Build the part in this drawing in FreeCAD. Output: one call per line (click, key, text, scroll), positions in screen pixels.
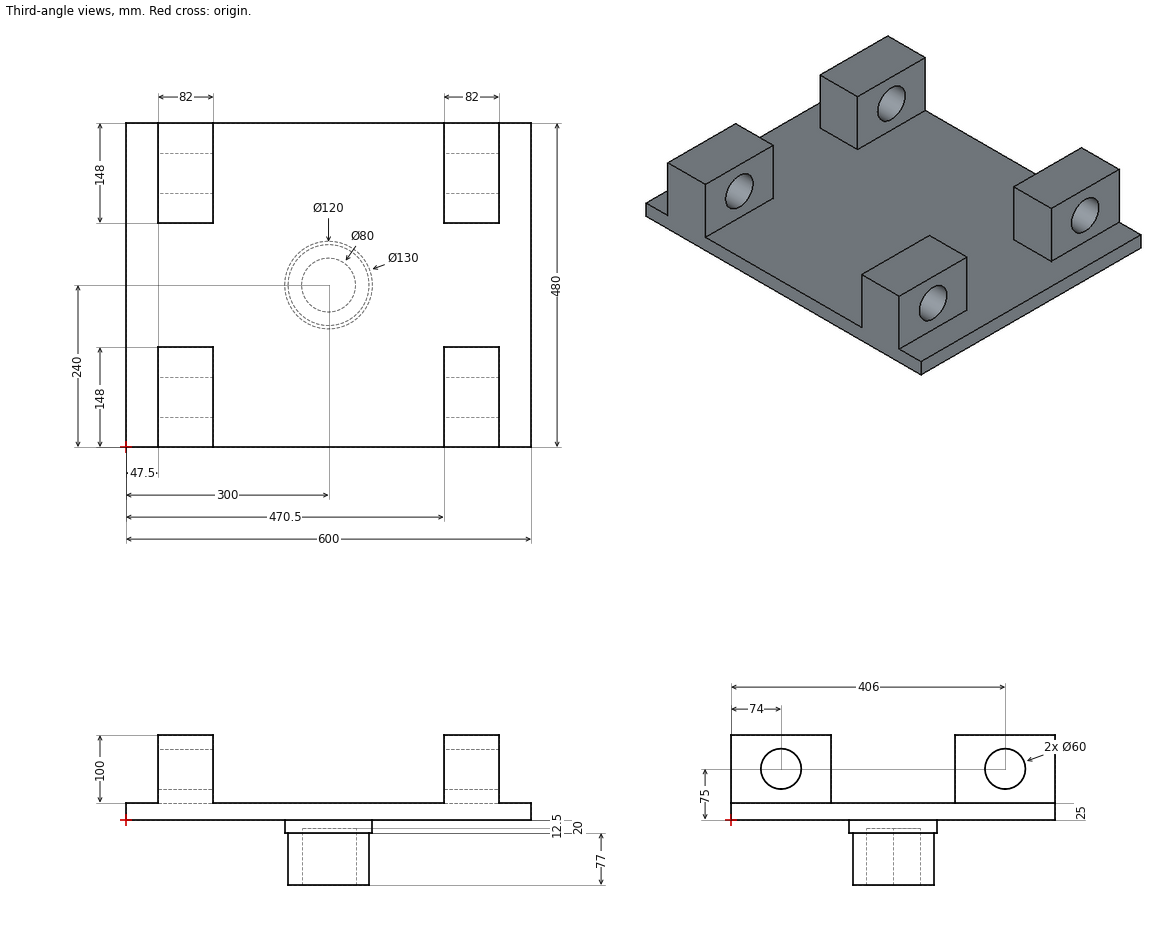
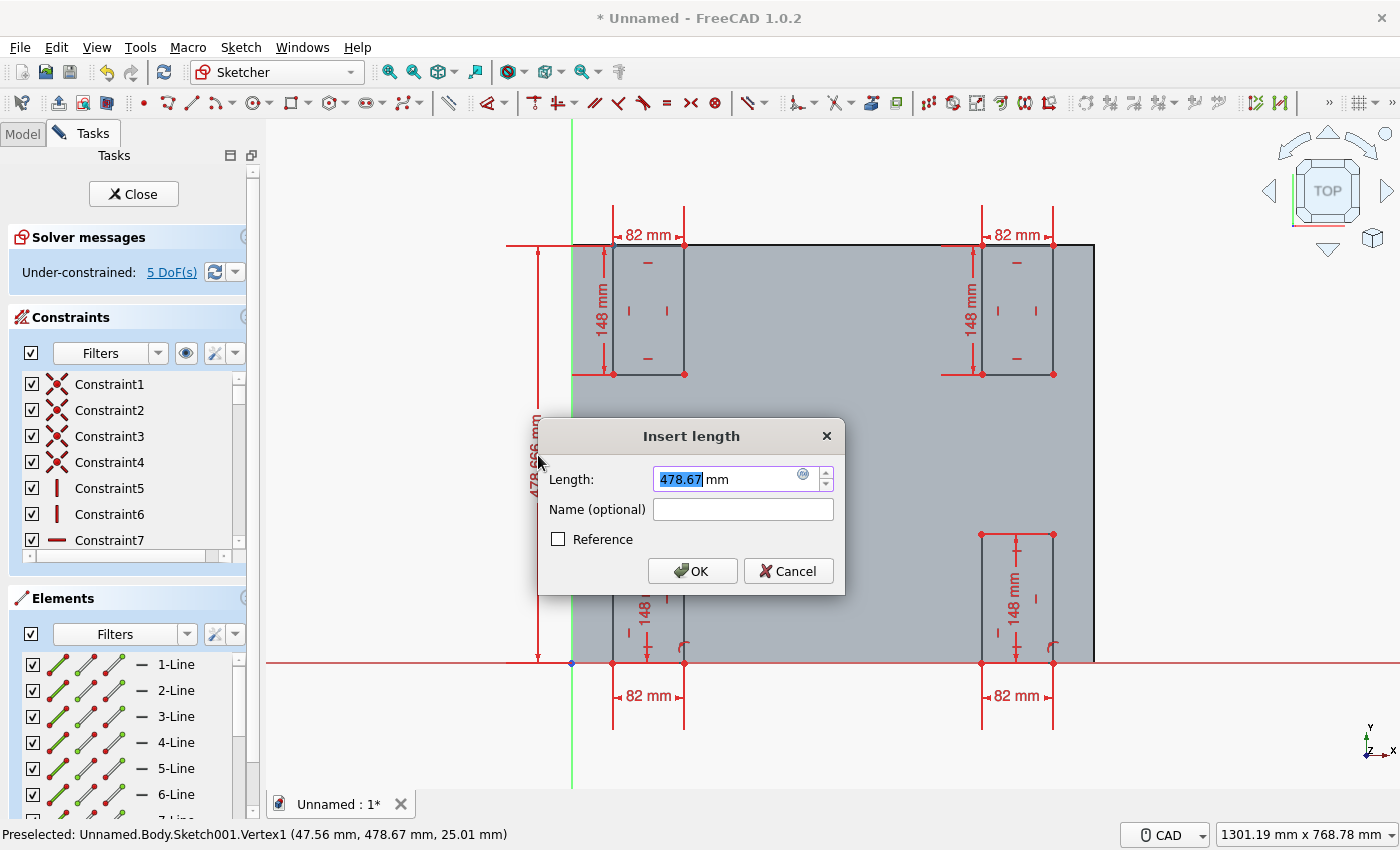
text(480)
key(Return)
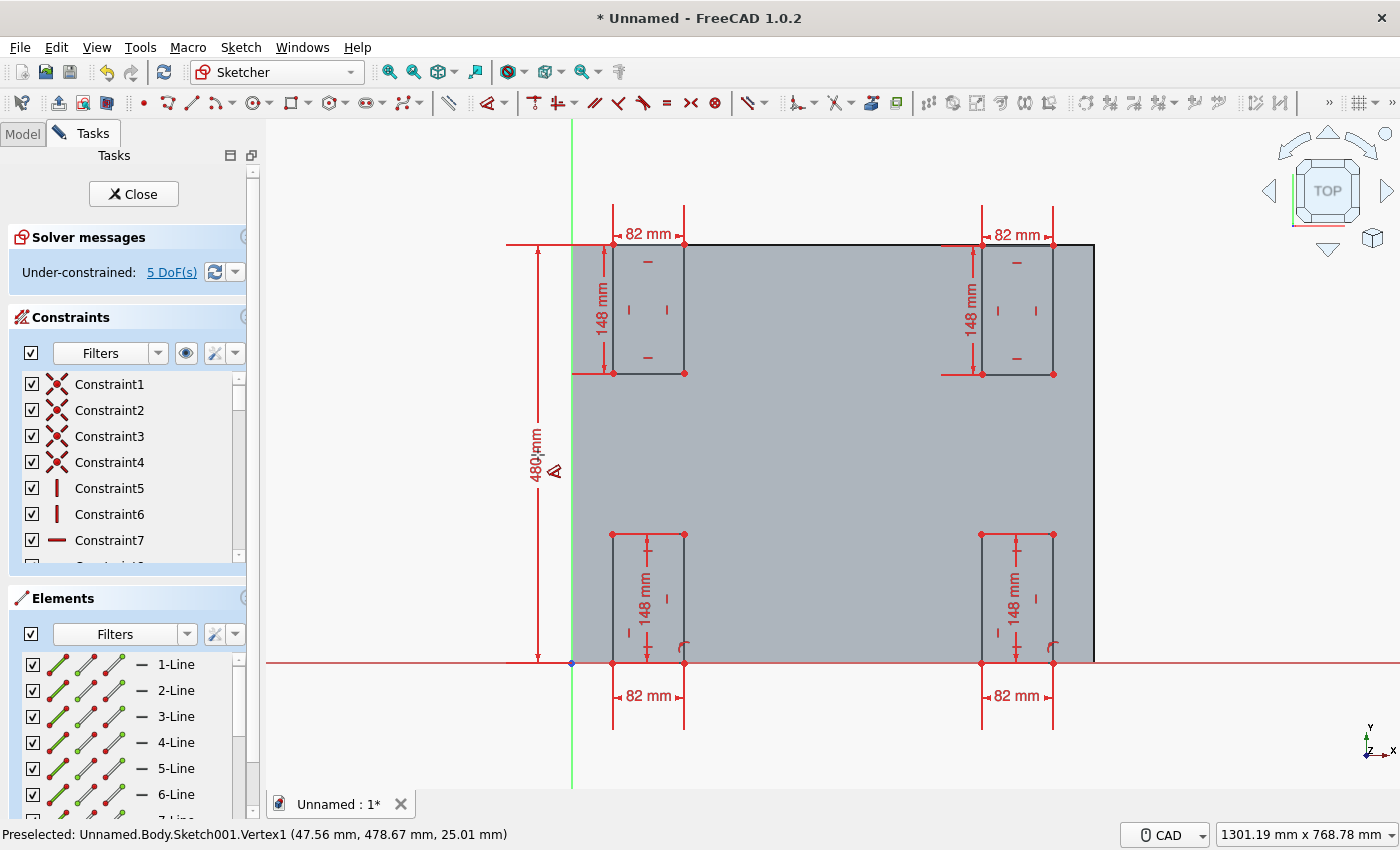
click(982, 246)
click(538, 359)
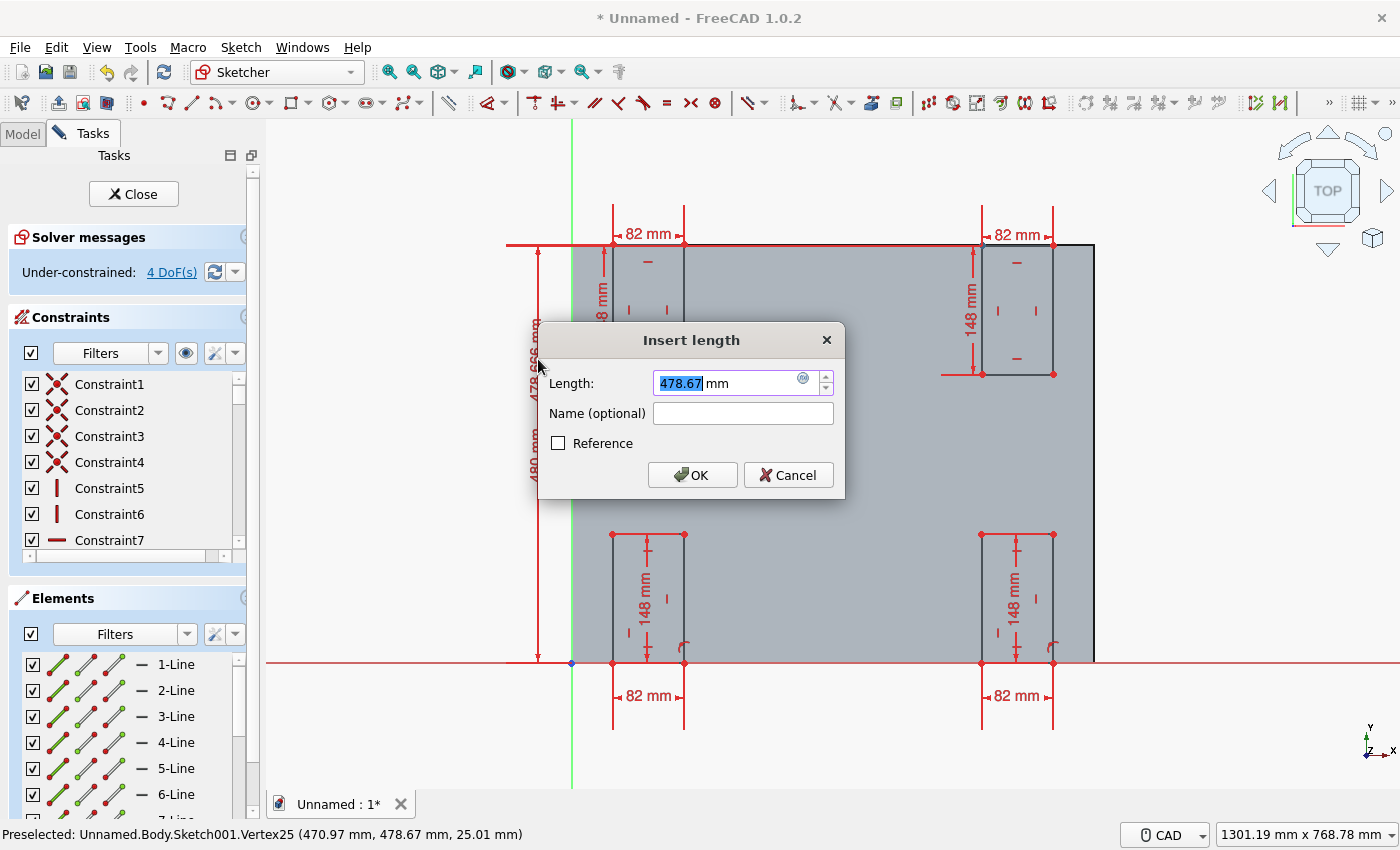
text(480)
key(Return)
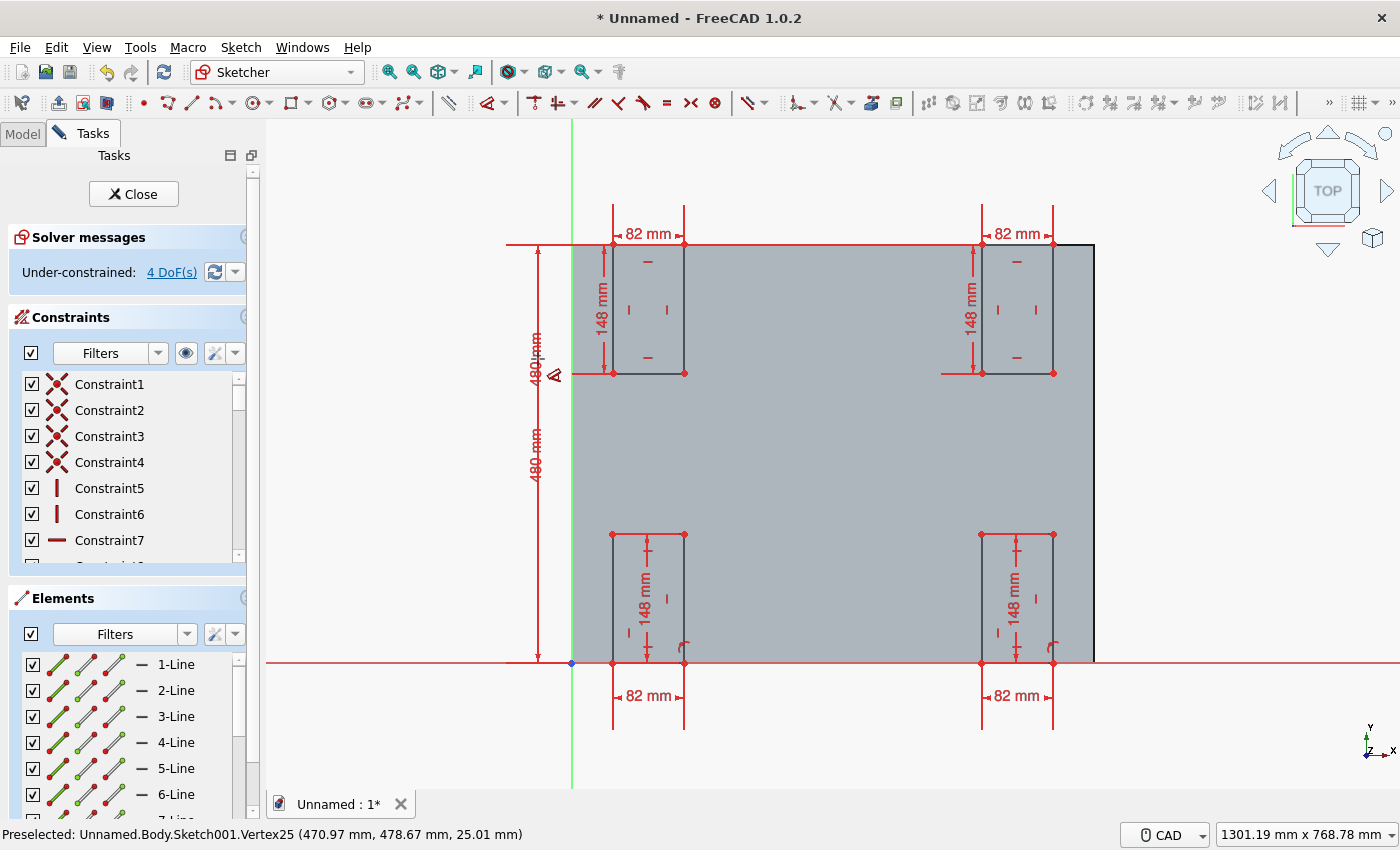
click(613, 245)
click(592, 211)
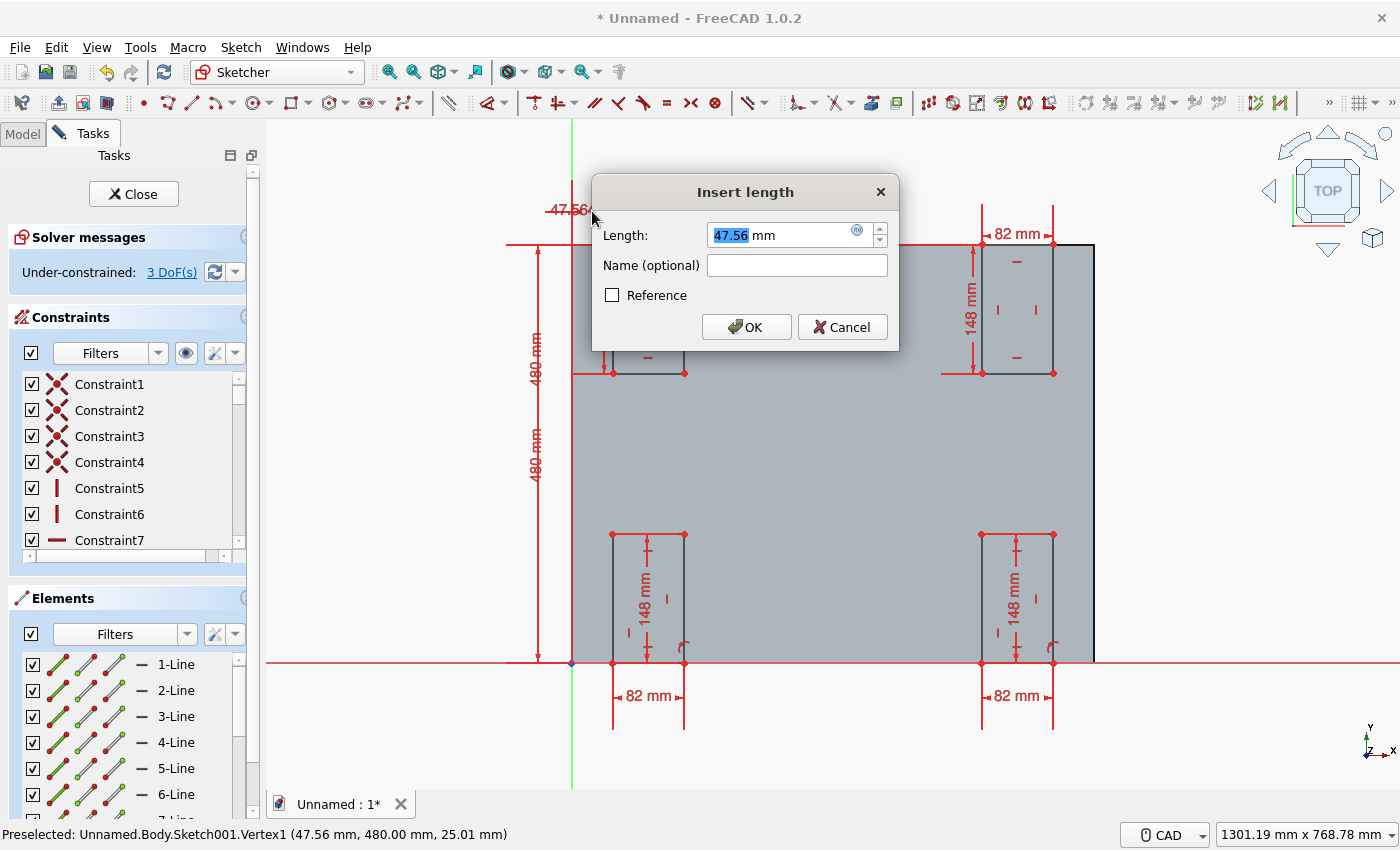
text(47.5)
key(Return)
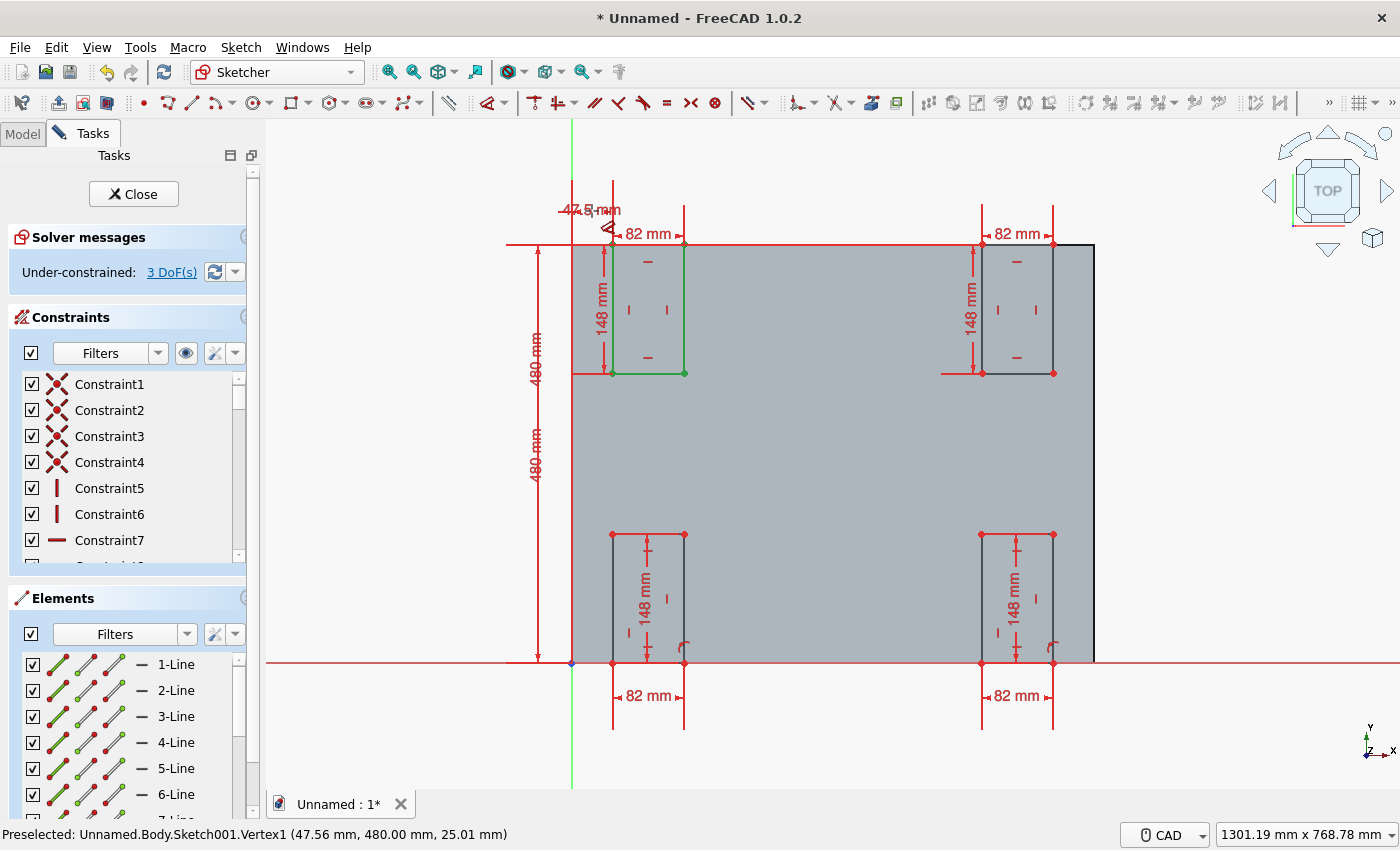
click(613, 534)
click(592, 500)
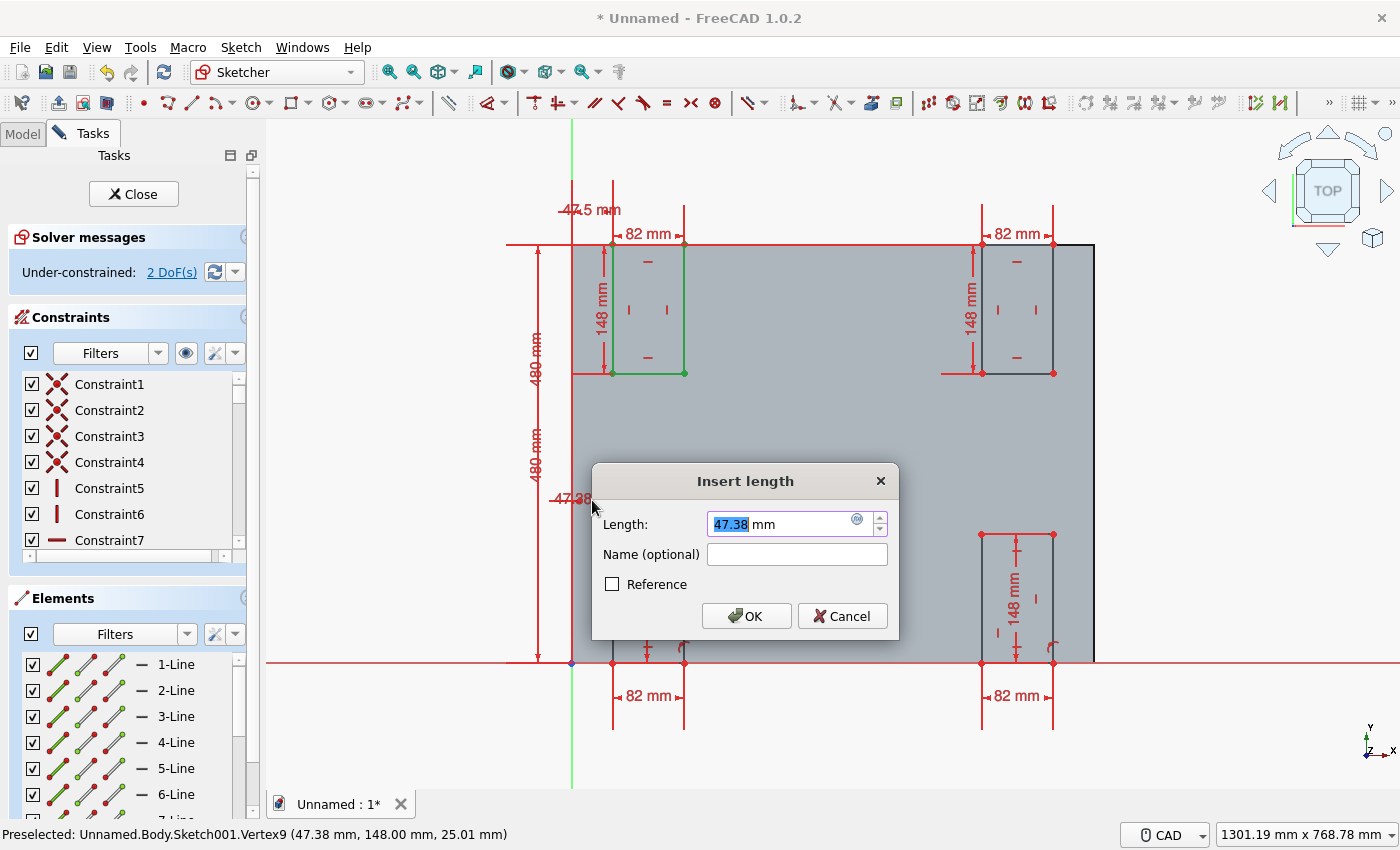
text(47.5)
key(Return)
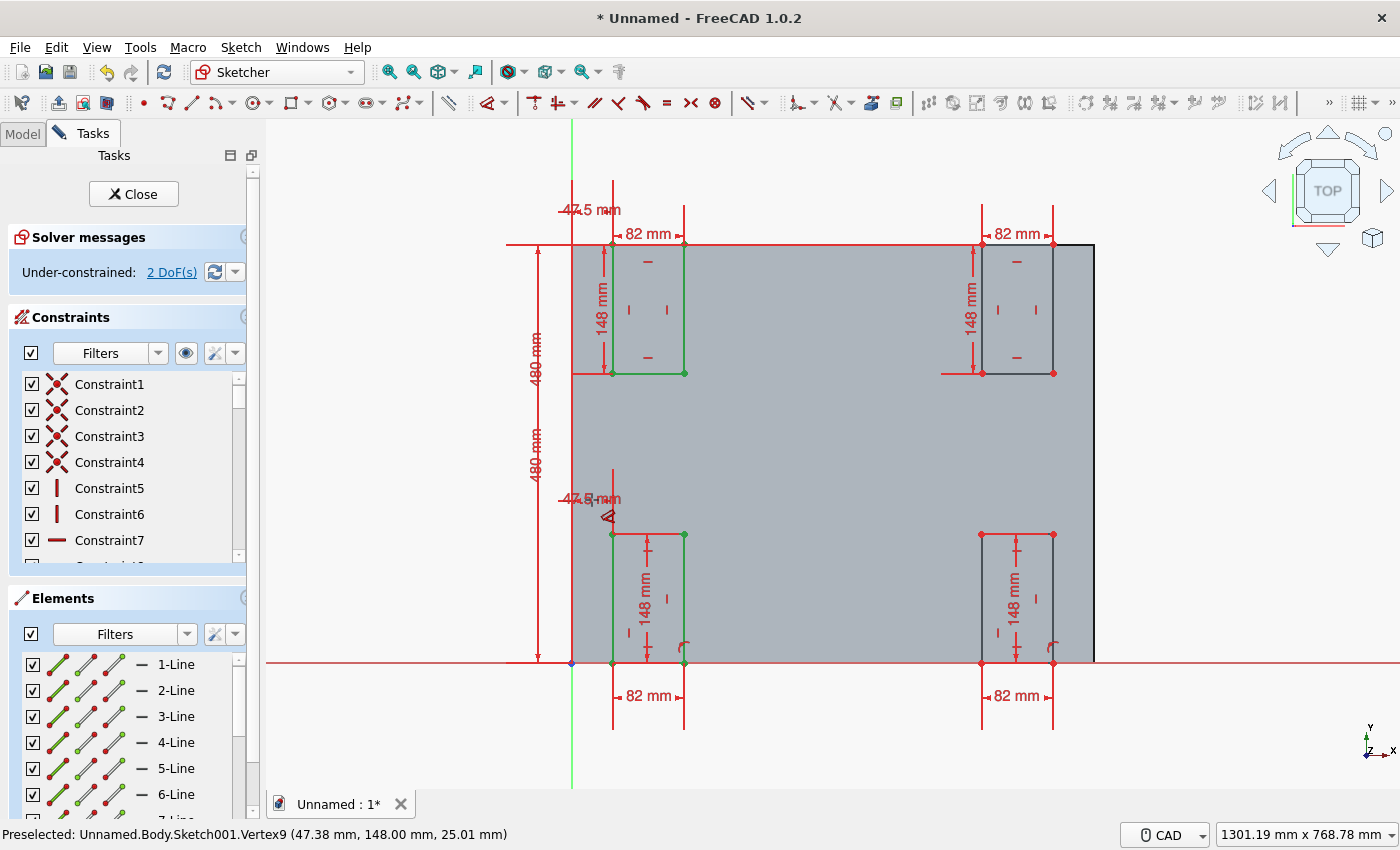
click(982, 534)
click(777, 697)